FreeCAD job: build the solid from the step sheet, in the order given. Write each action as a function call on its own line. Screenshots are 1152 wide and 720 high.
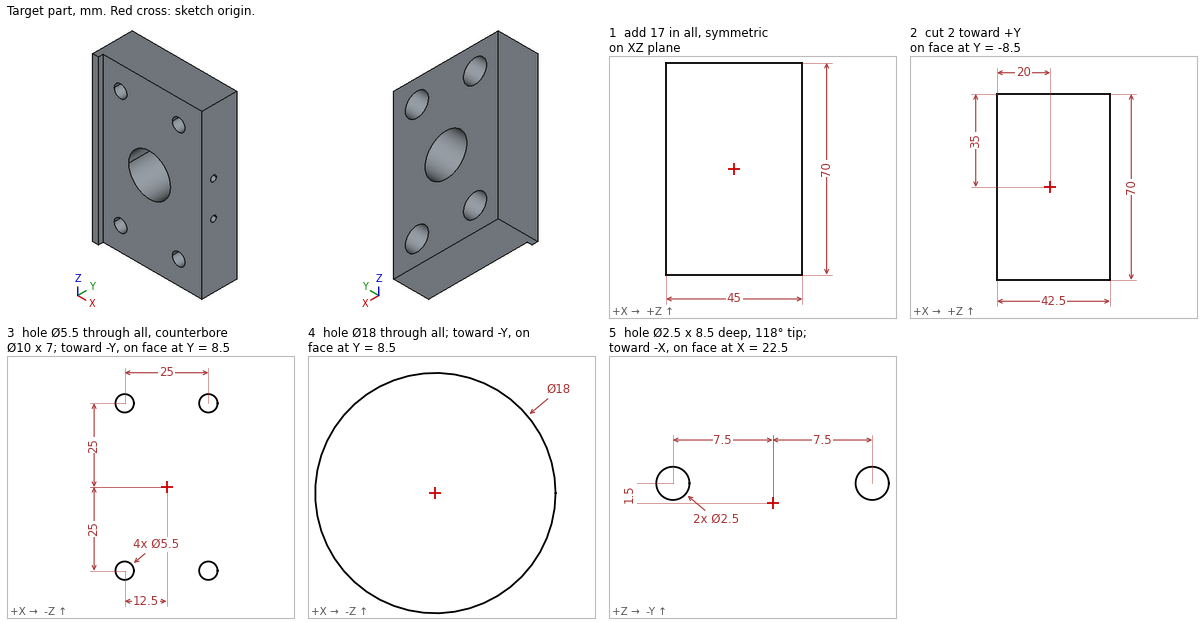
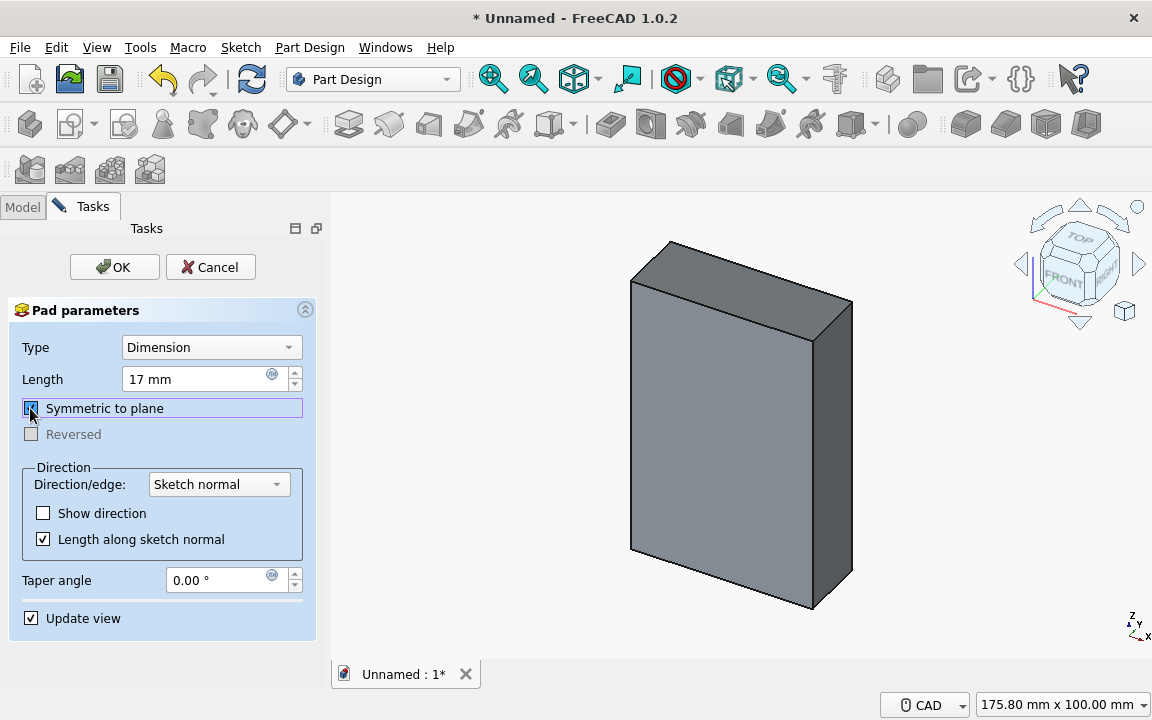
click(115, 267)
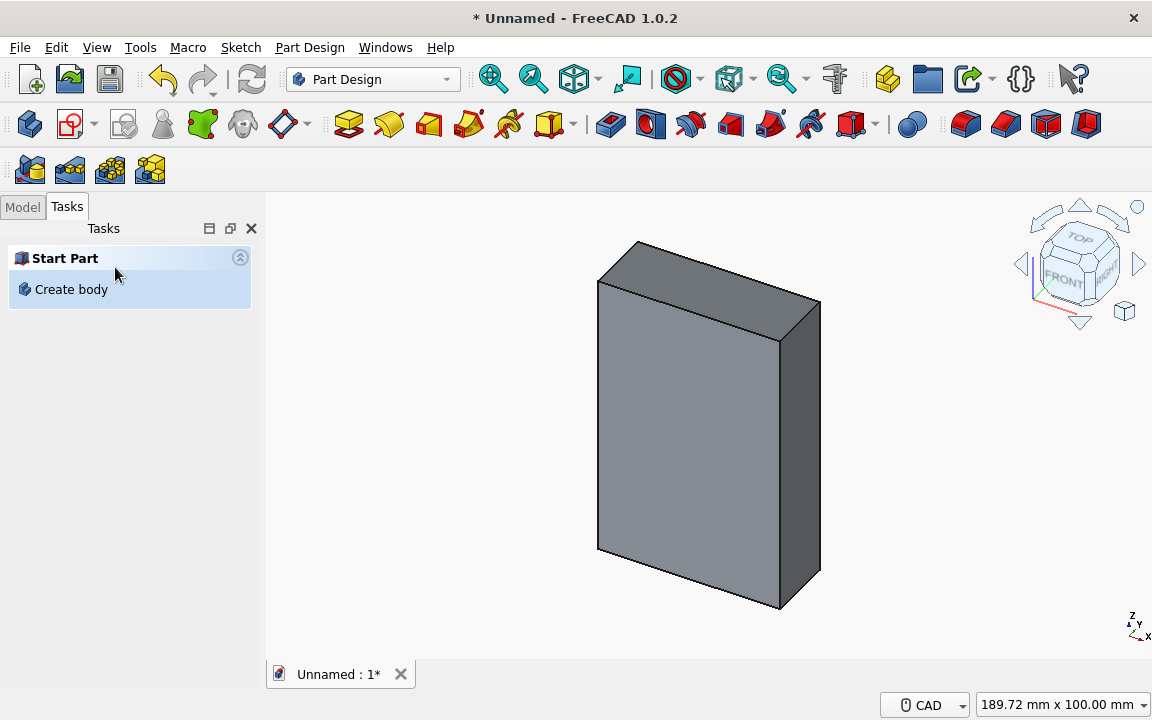
click(689, 406)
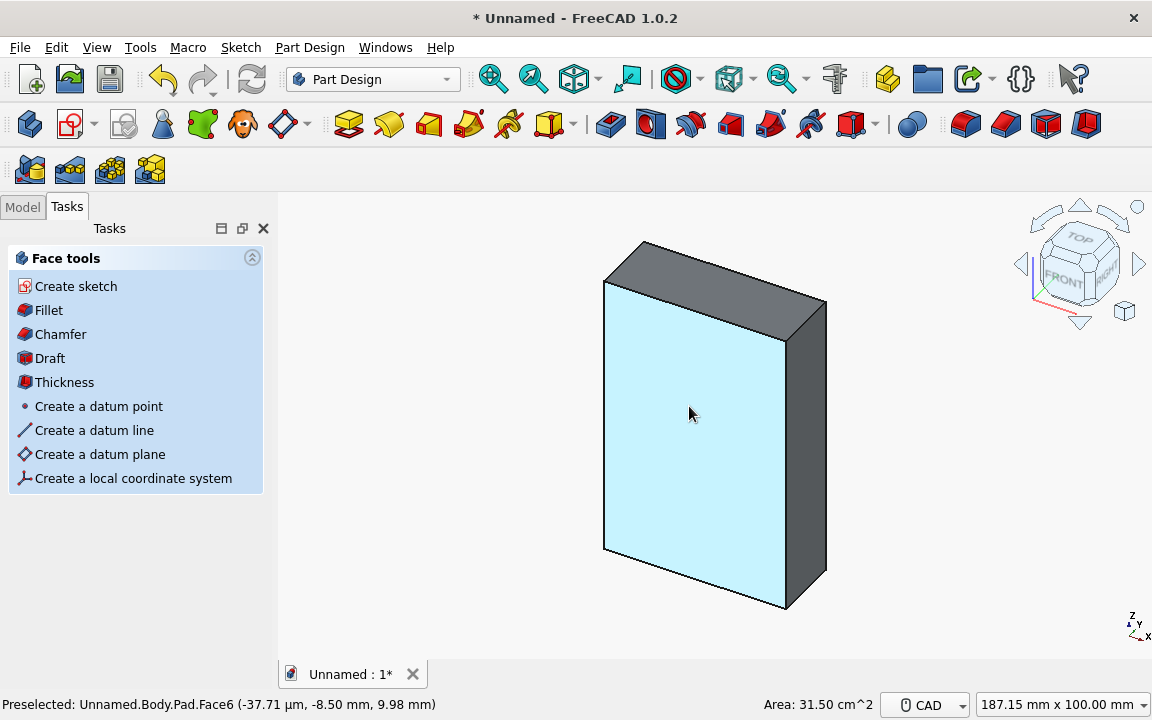
click(70, 124)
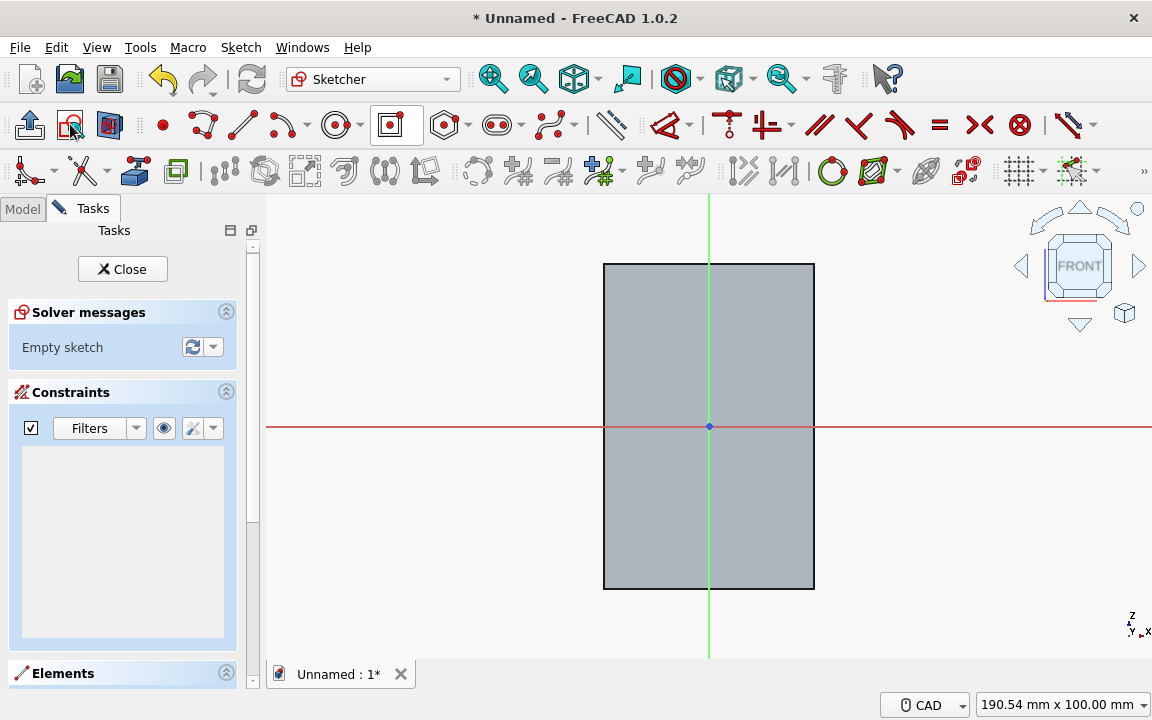
click(418, 126)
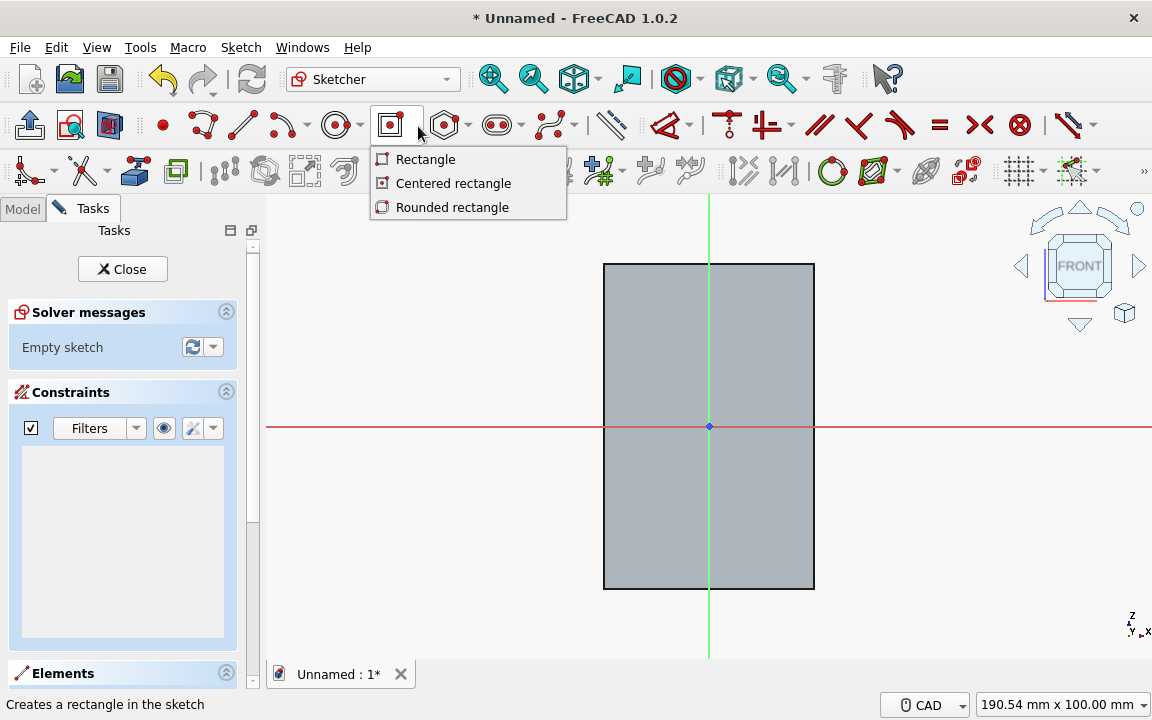
click(468, 159)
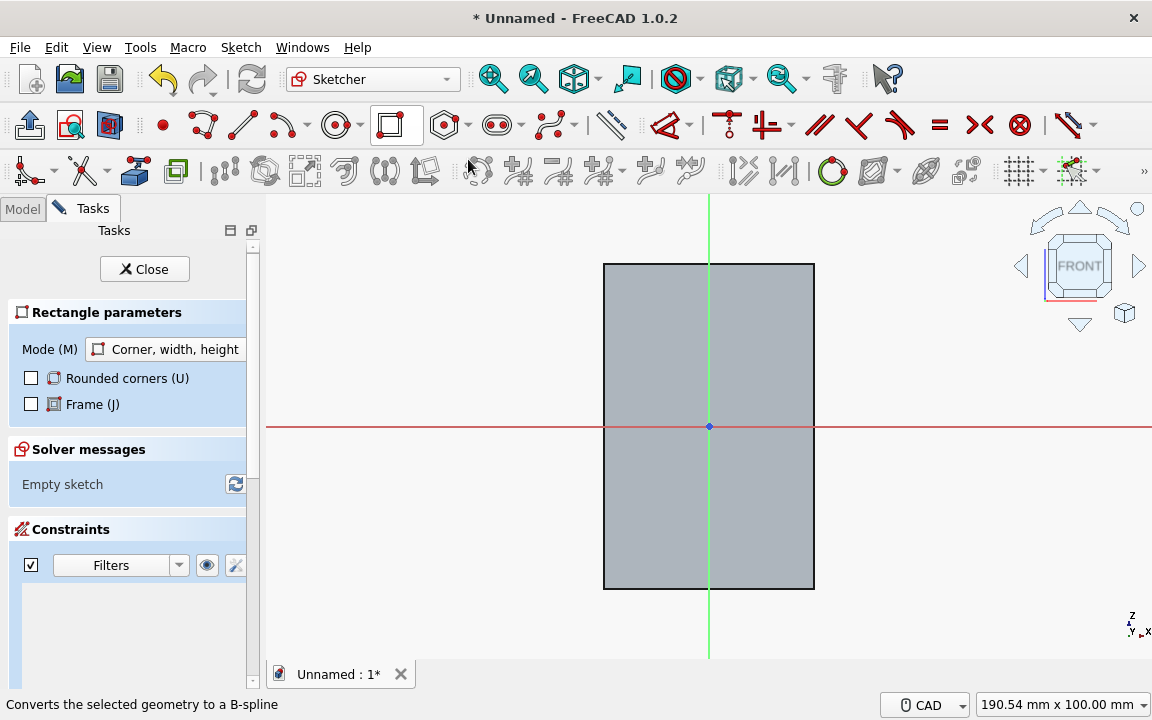
click(616, 264)
move(814, 589)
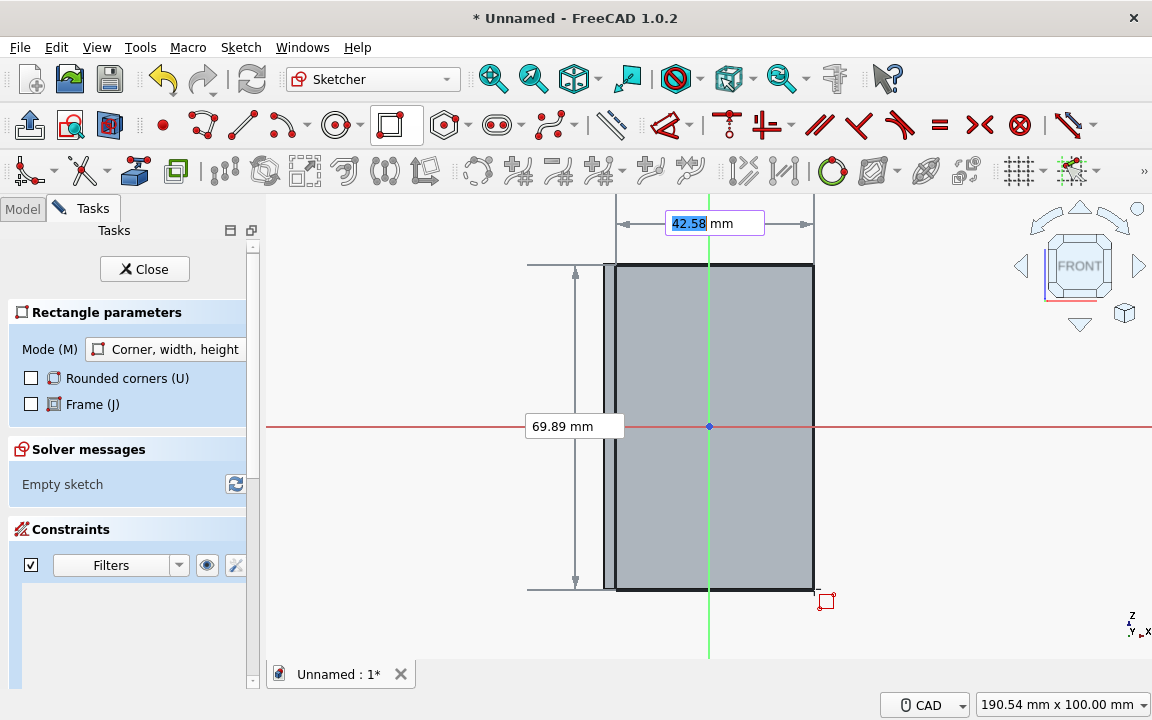
text(42.5)
key(Tab)
text(70)
key(Return)
key(Escape)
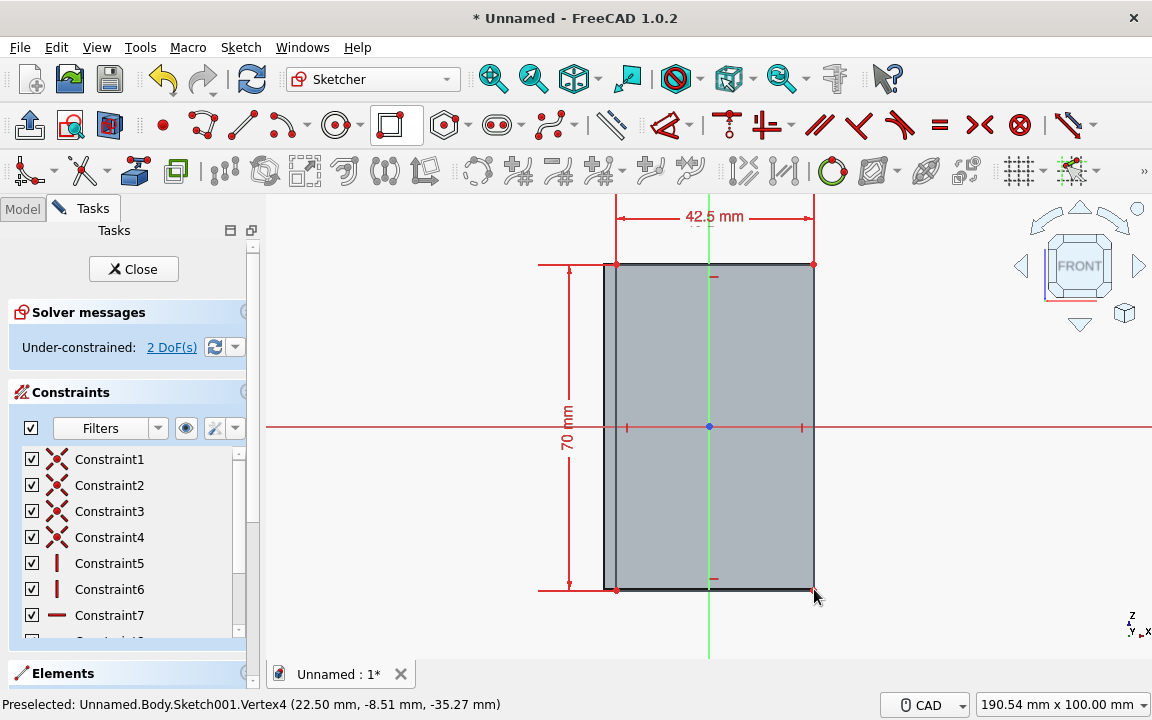
click(666, 126)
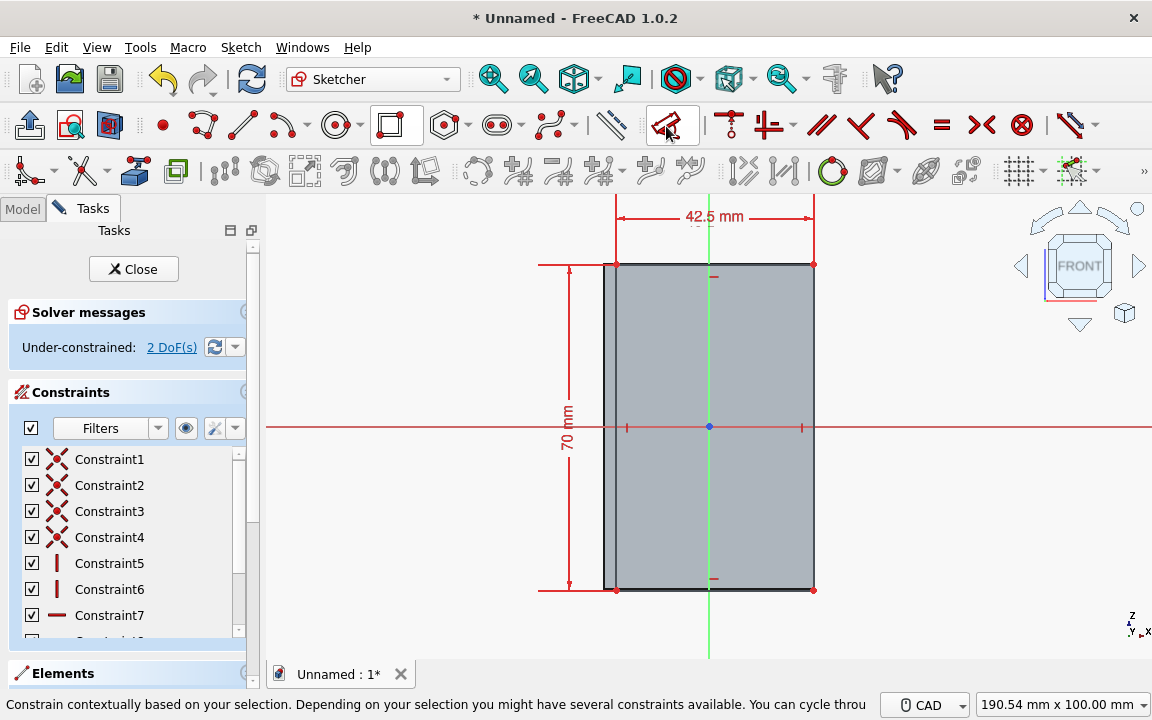
click(616, 265)
click(662, 231)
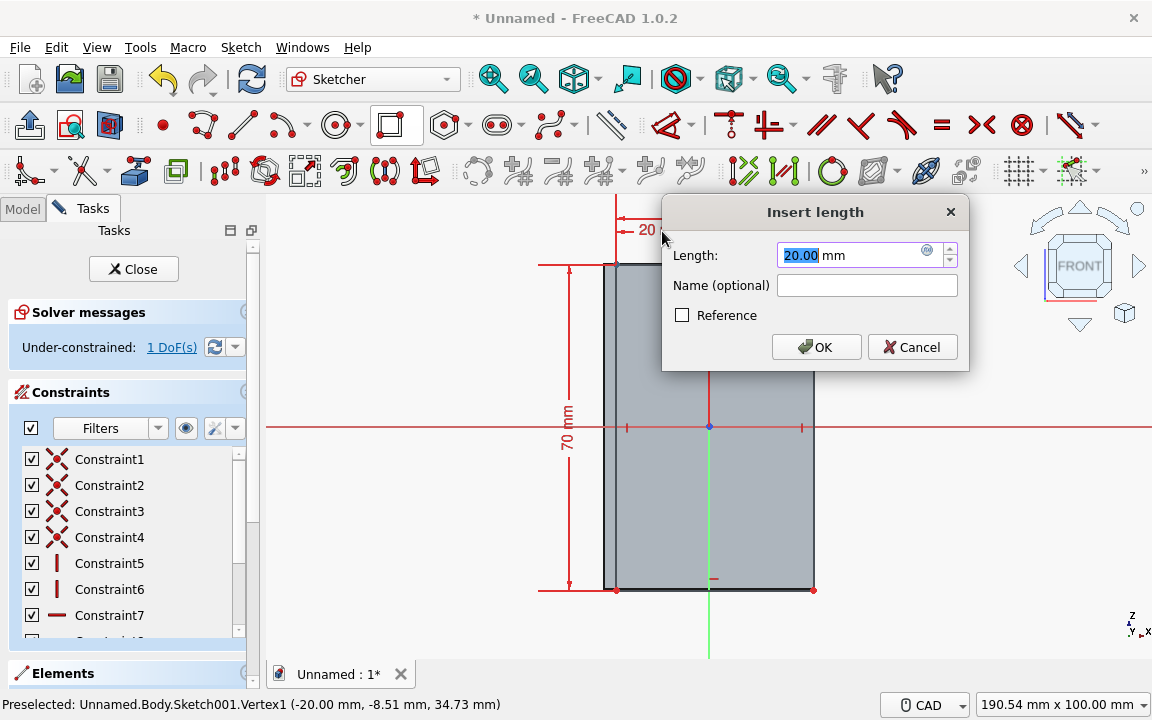
text(20)
key(Return)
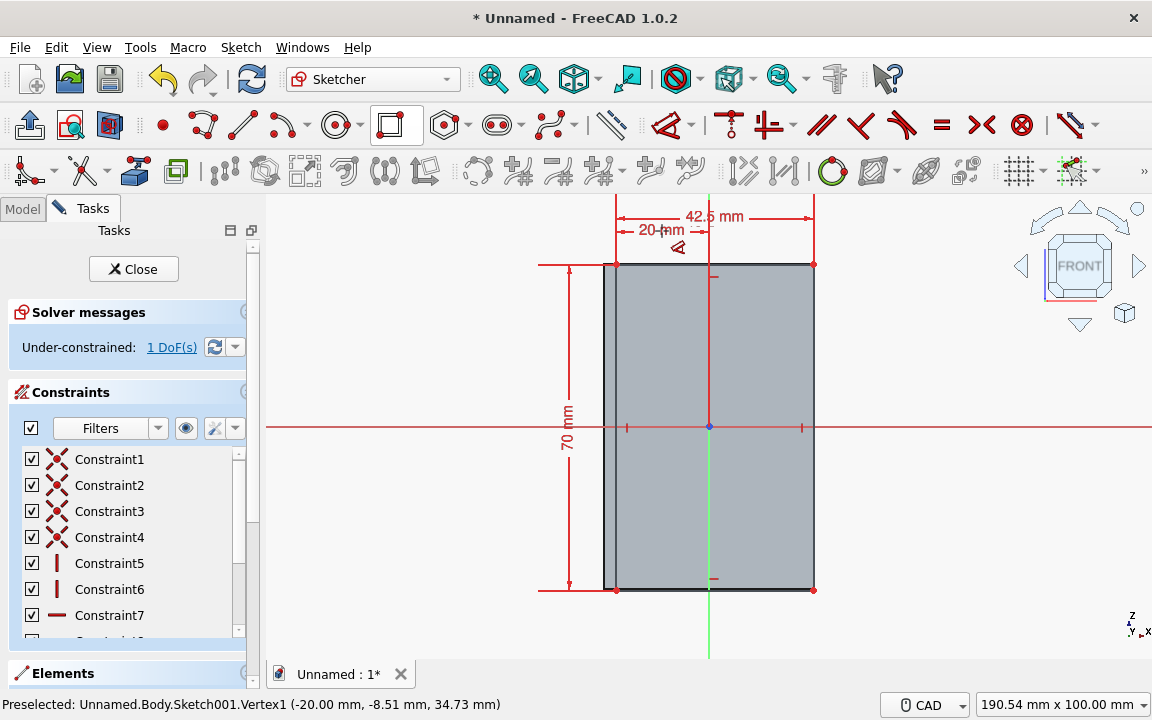
click(616, 265)
click(582, 346)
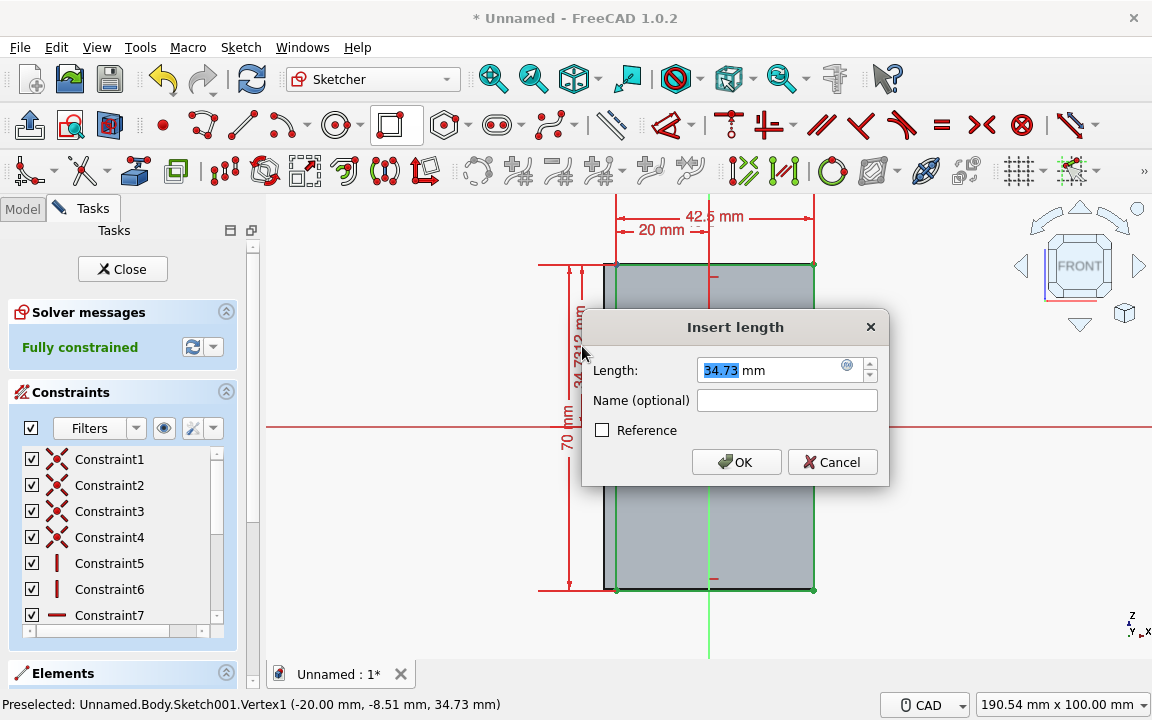
text(35)
key(Return)
key(Escape)